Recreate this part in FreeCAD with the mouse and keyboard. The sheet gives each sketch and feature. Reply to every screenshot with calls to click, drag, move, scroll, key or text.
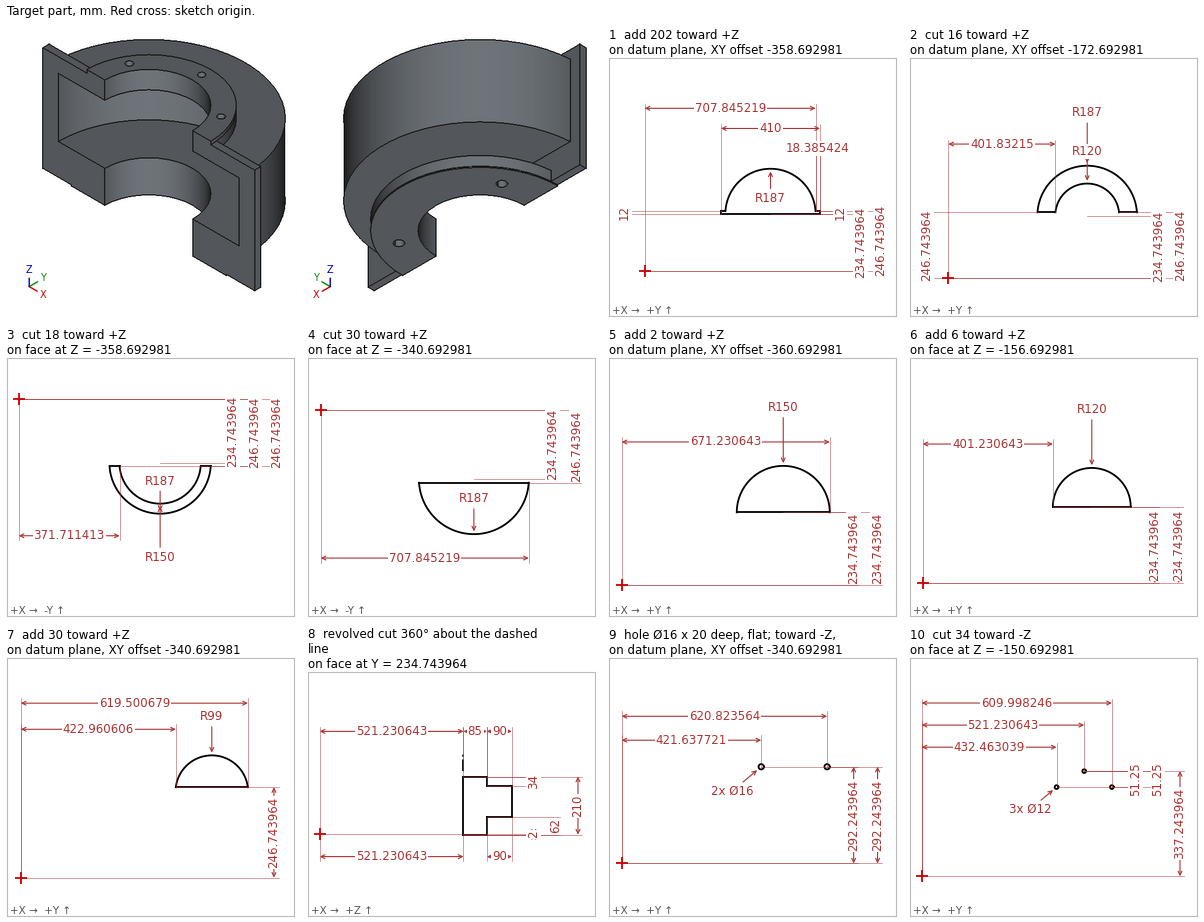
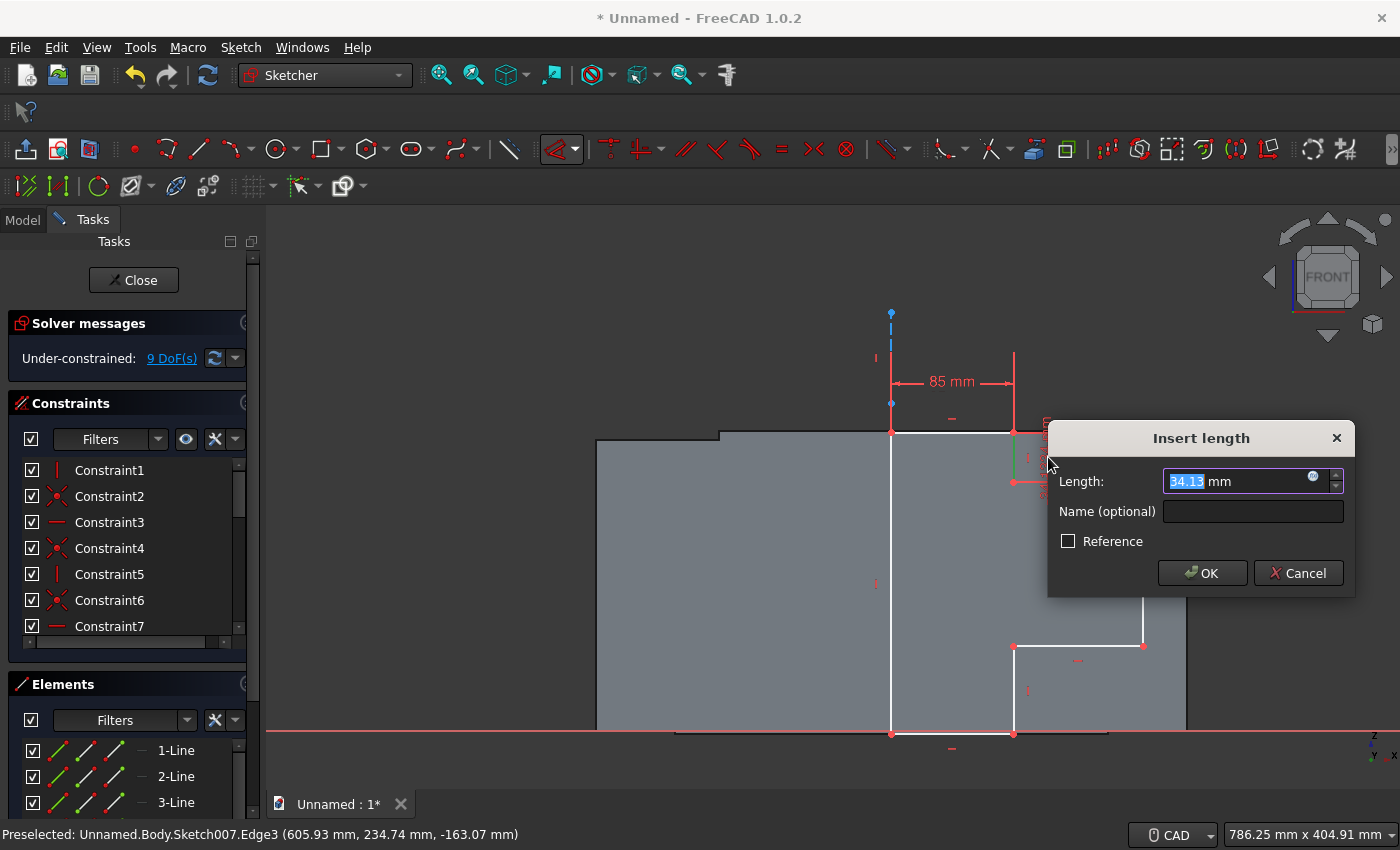
text(34)
key(Return)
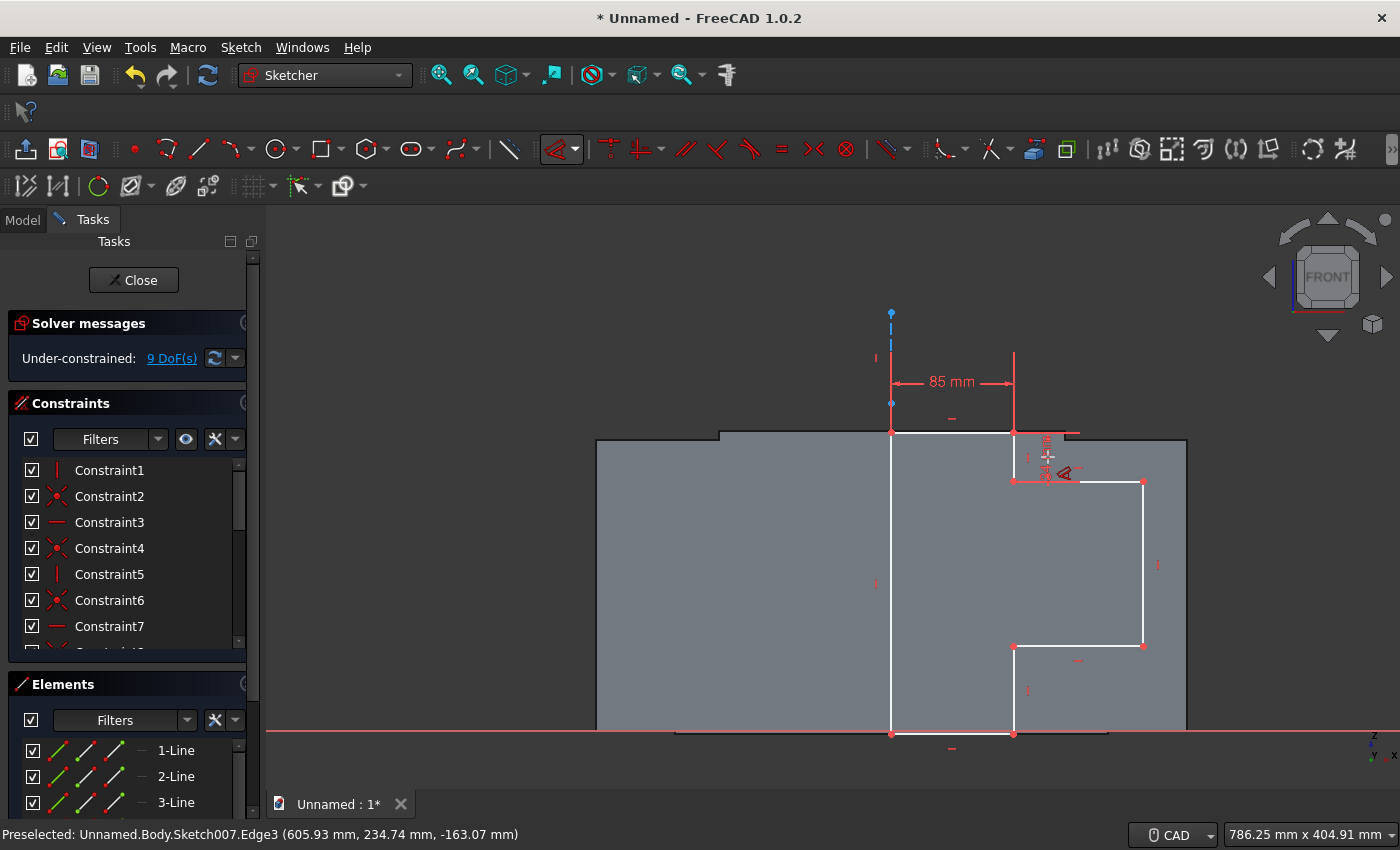
click(1053, 482)
click(1124, 448)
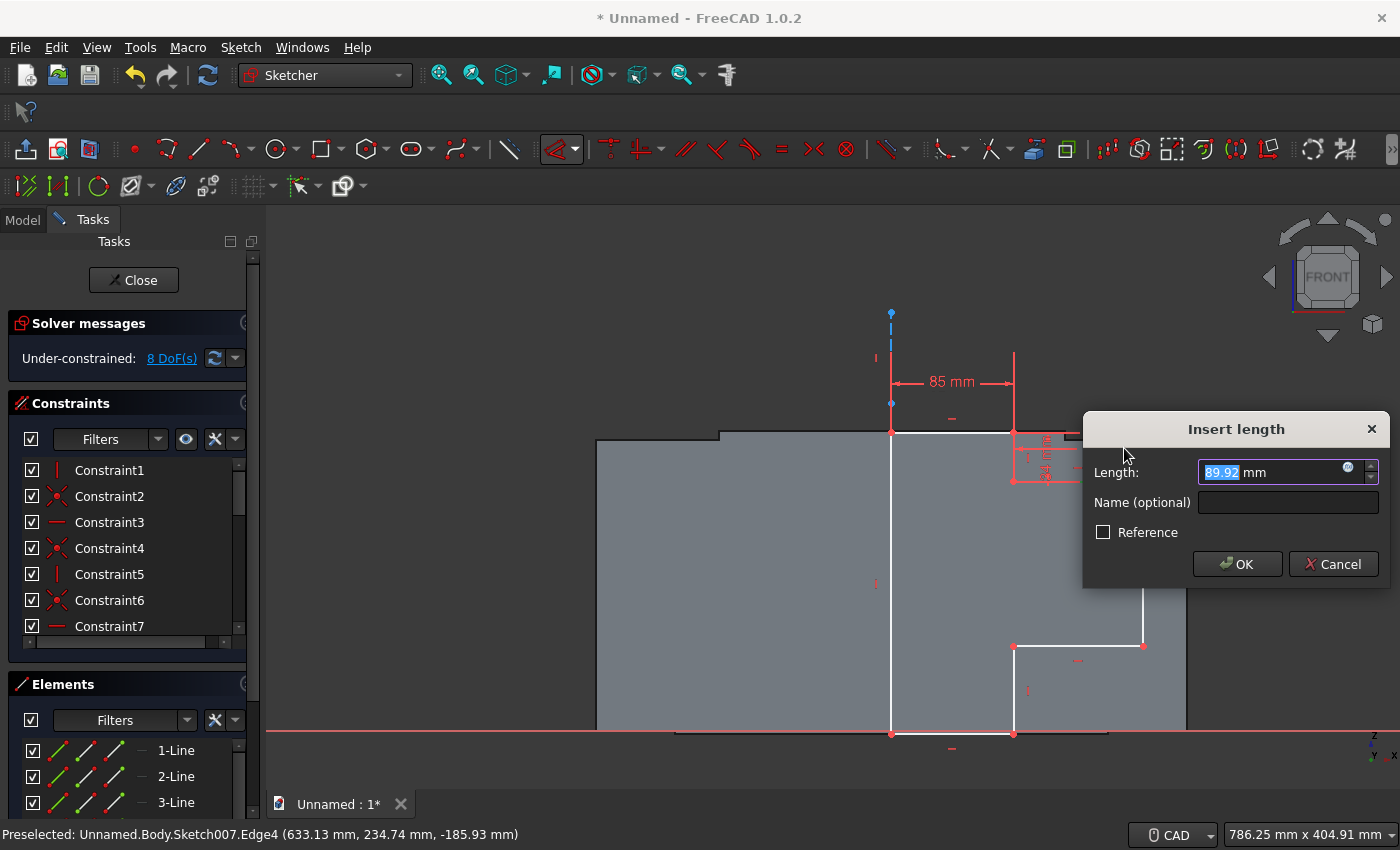
text(90)
key(Return)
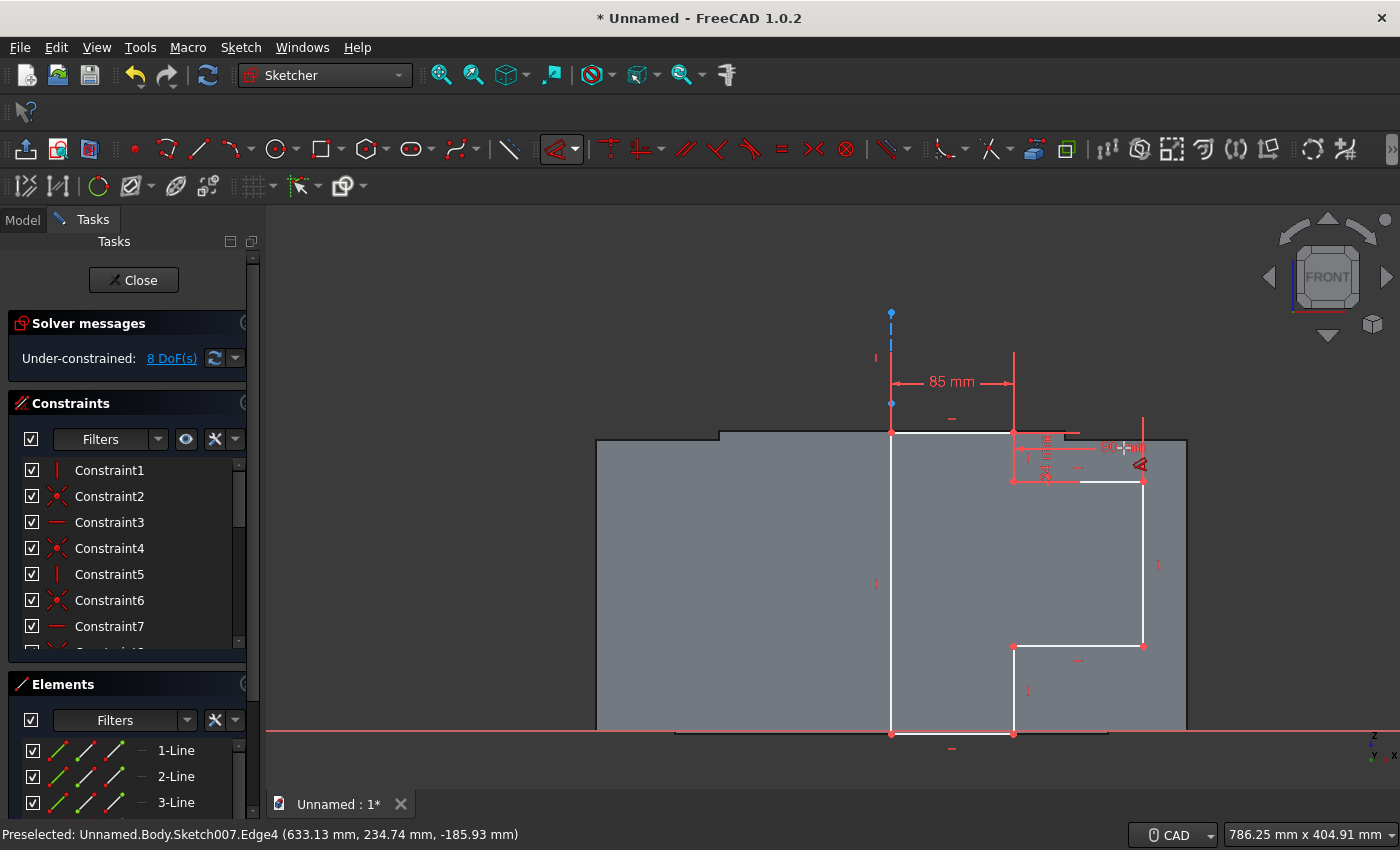
click(1105, 646)
click(1079, 680)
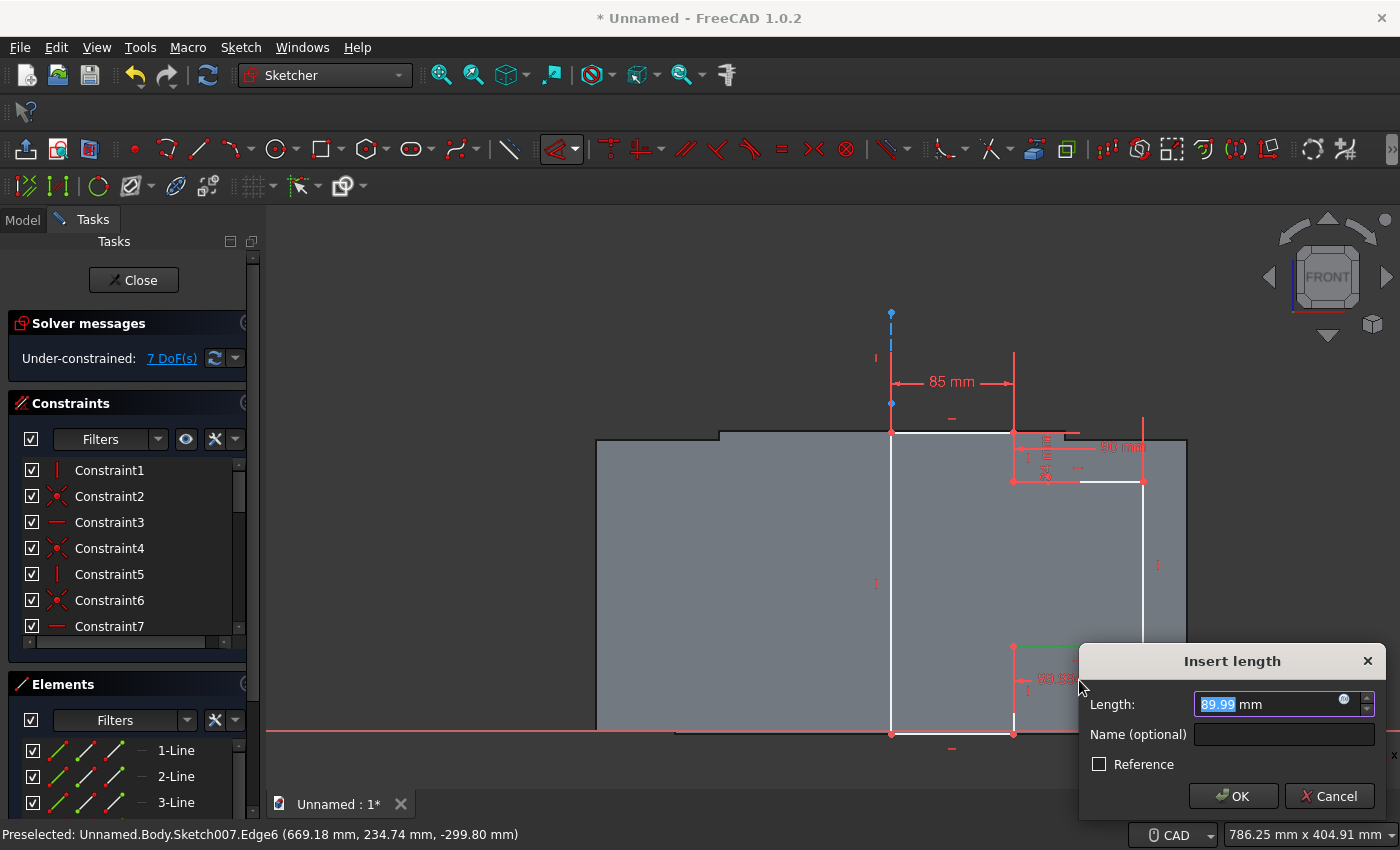
text(90)
key(Return)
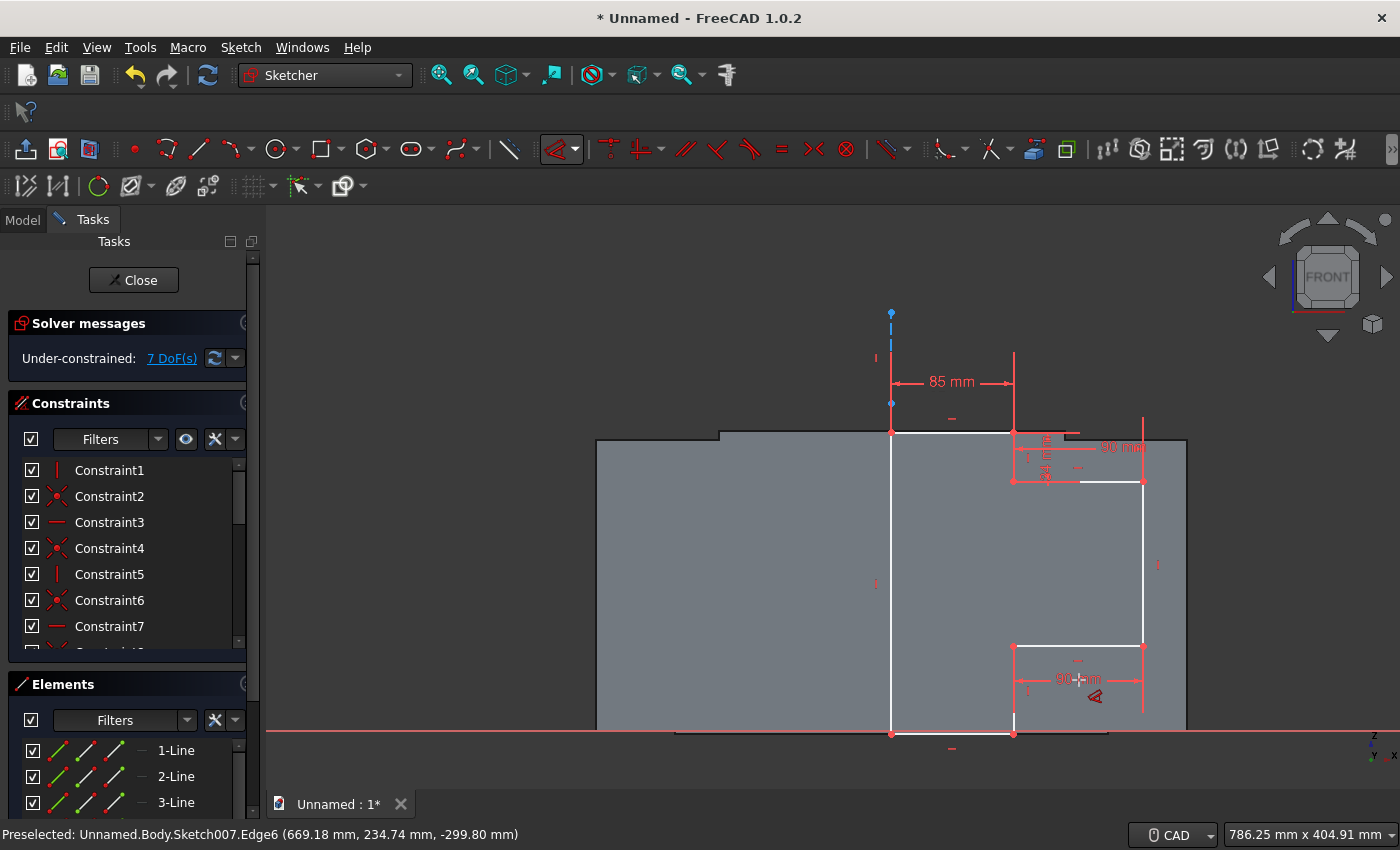
click(1014, 673)
click(1048, 710)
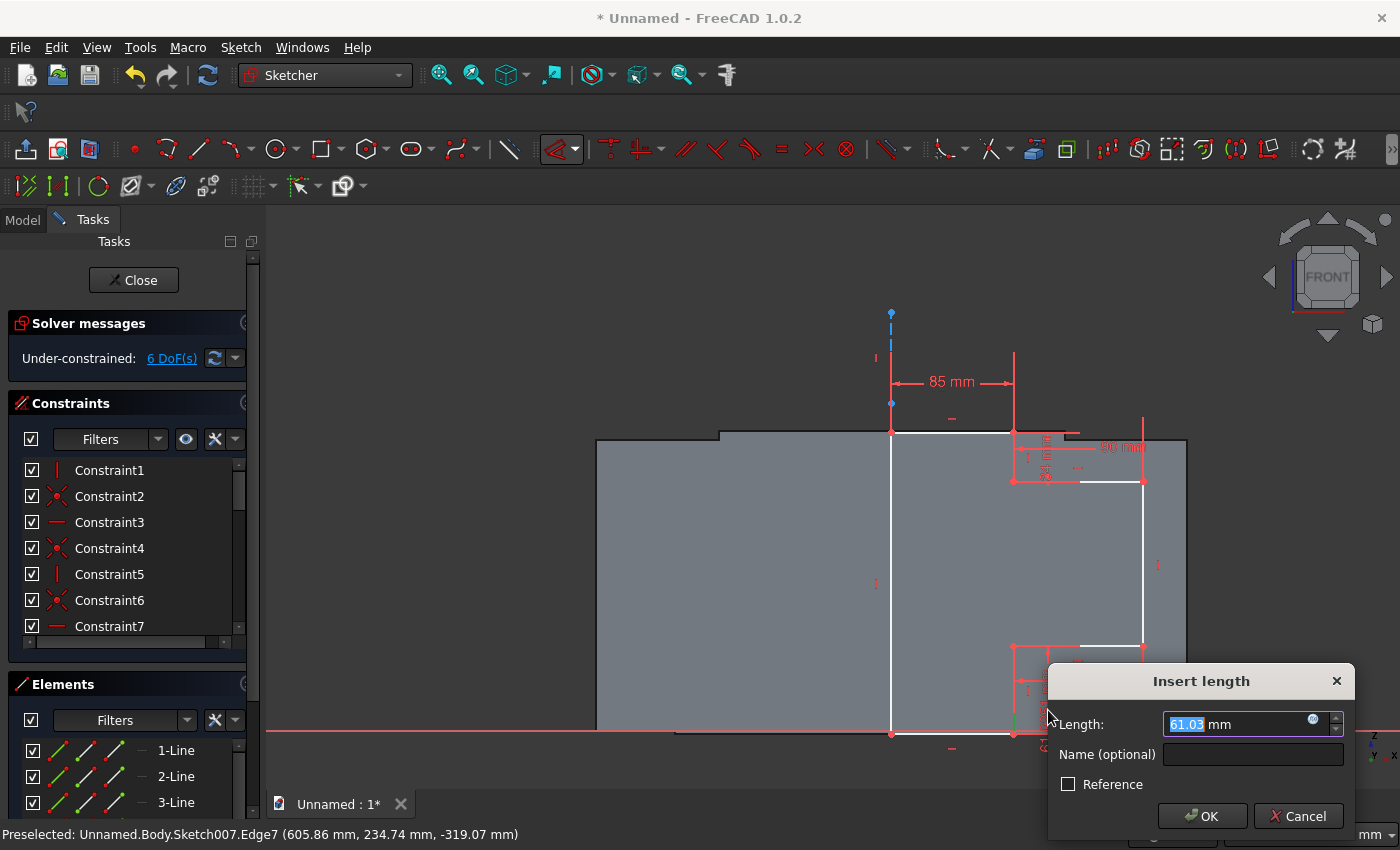
text(62)
key(Return)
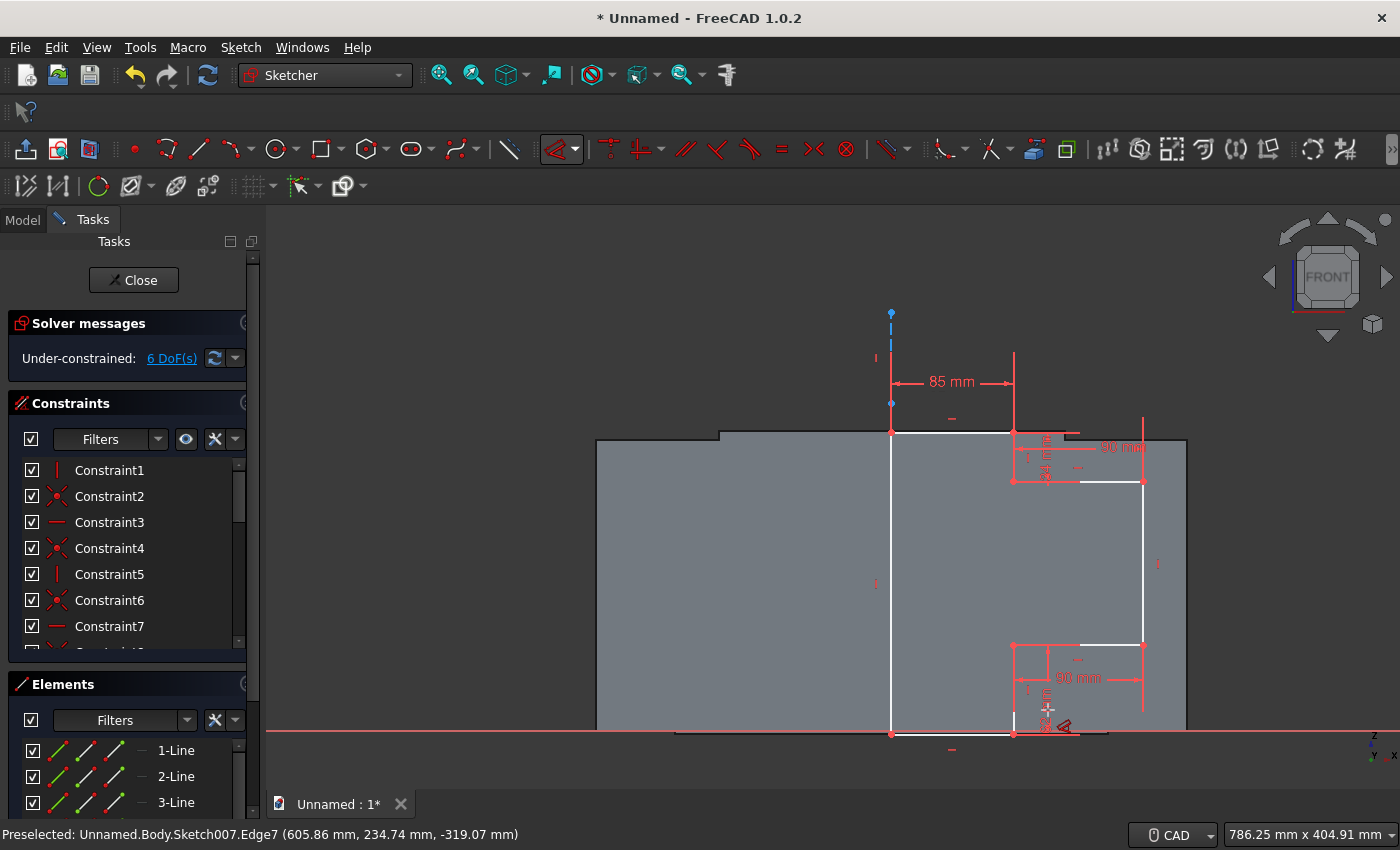
scroll(891, 735, up, 14)